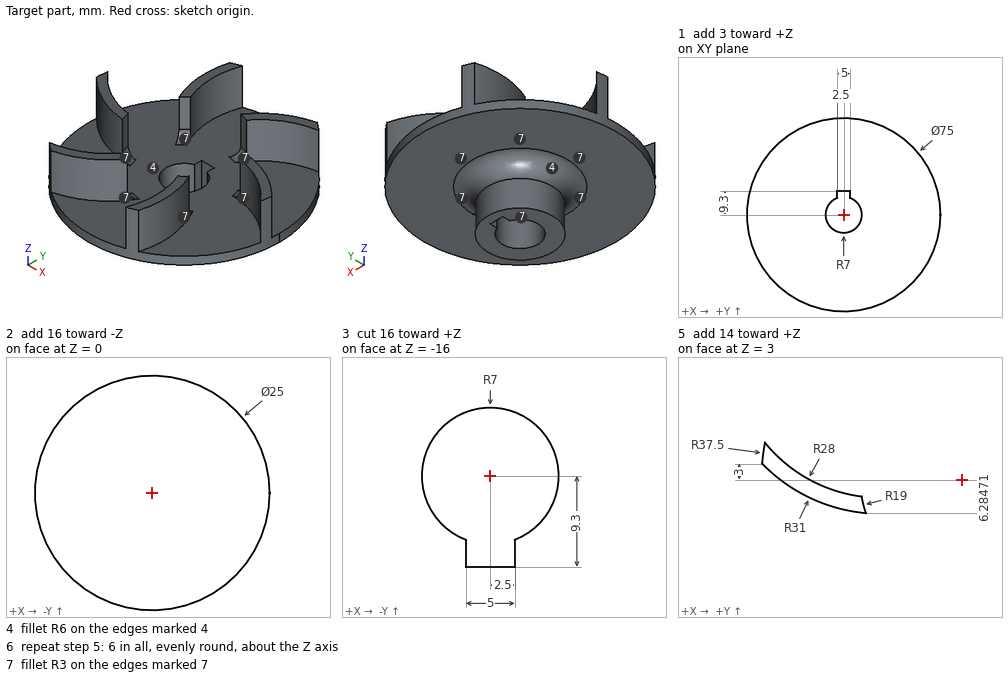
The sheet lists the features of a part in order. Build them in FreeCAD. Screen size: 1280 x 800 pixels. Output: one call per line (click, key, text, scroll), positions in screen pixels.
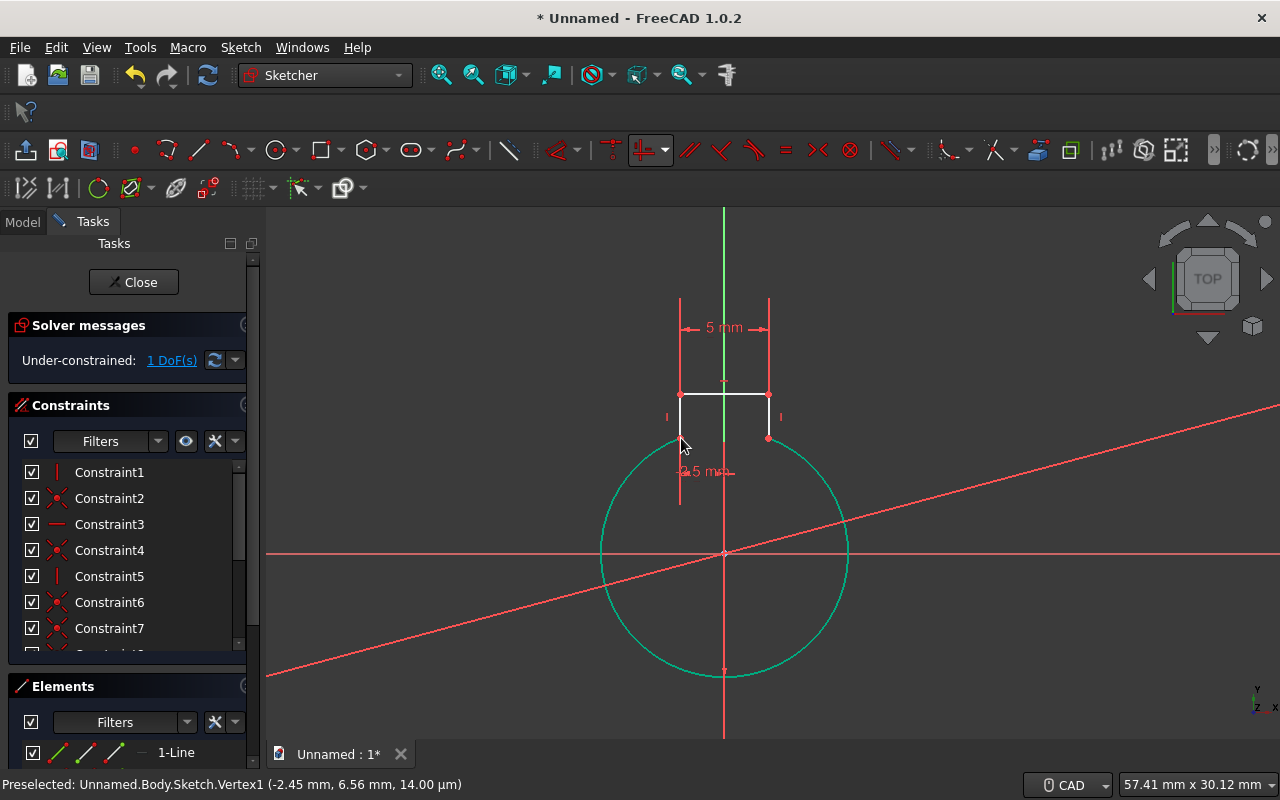
click(680, 394)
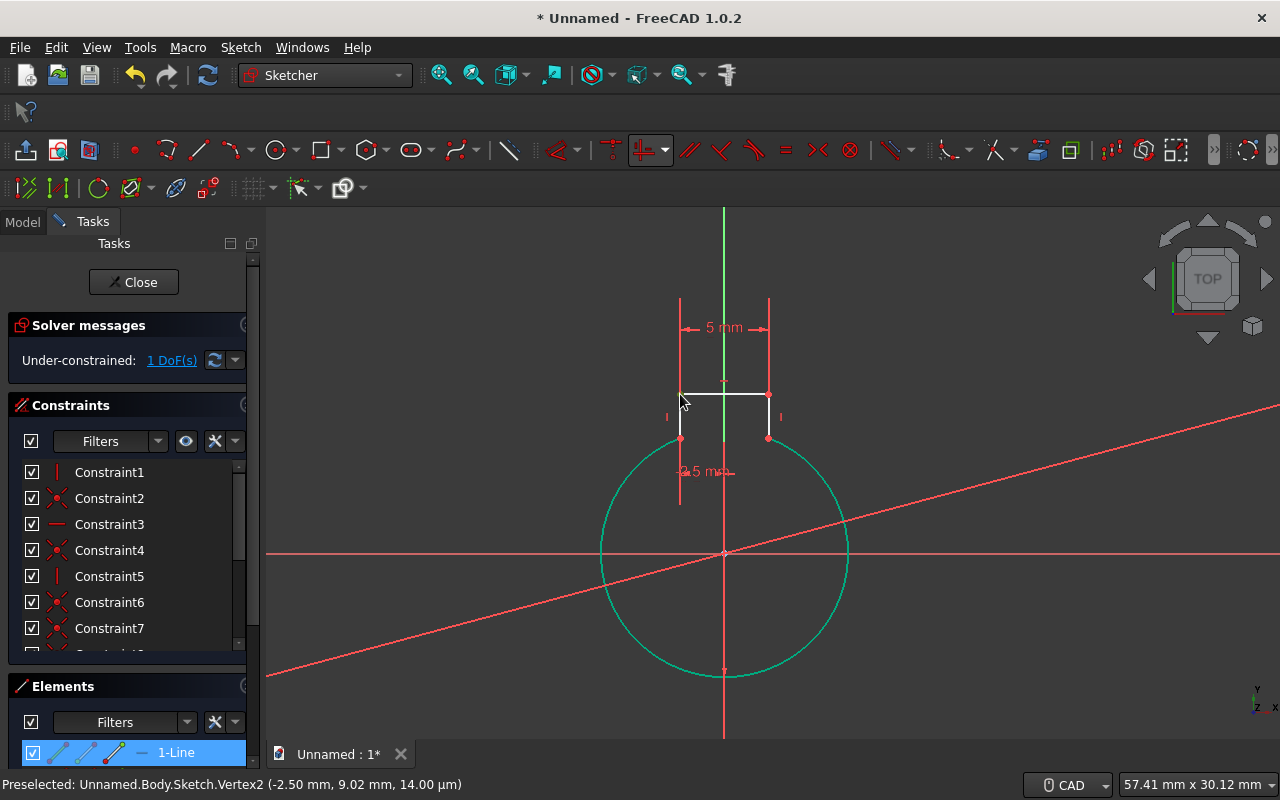
key(i)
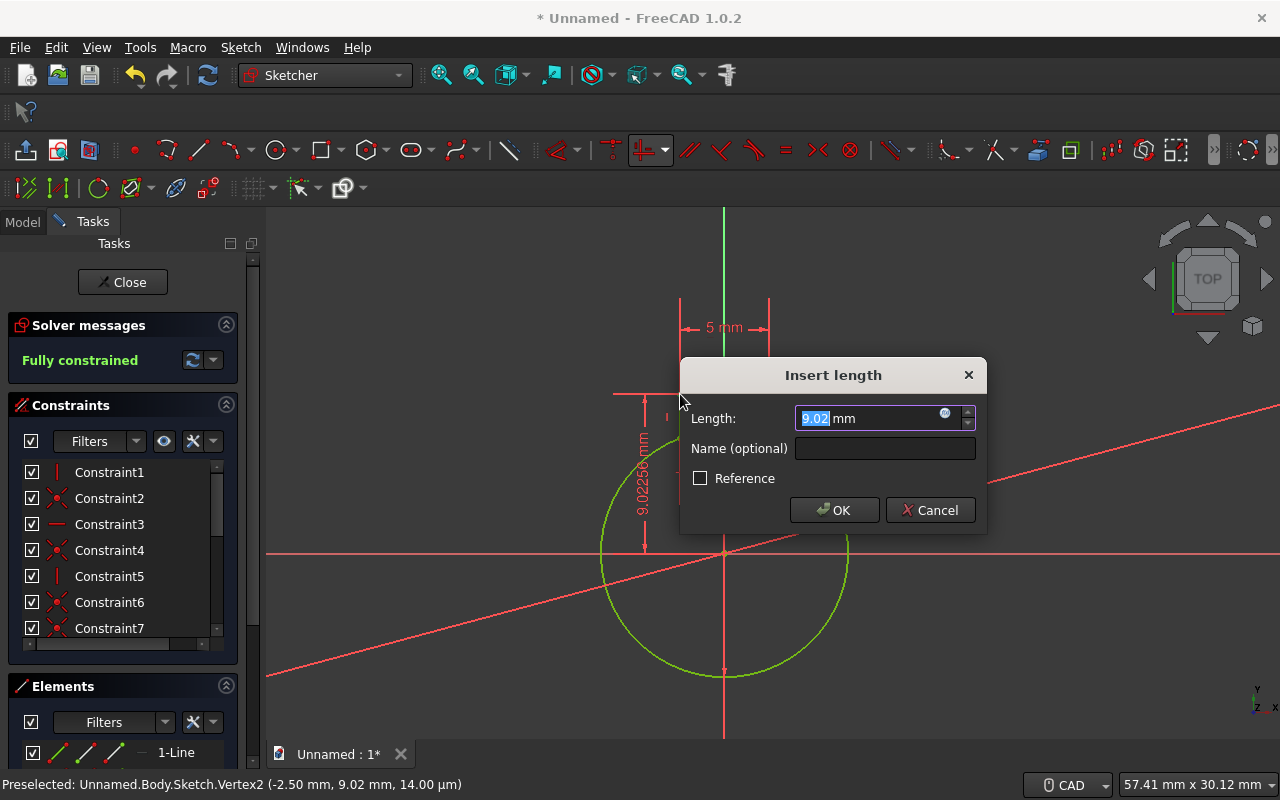
text(9.3)
key(Return)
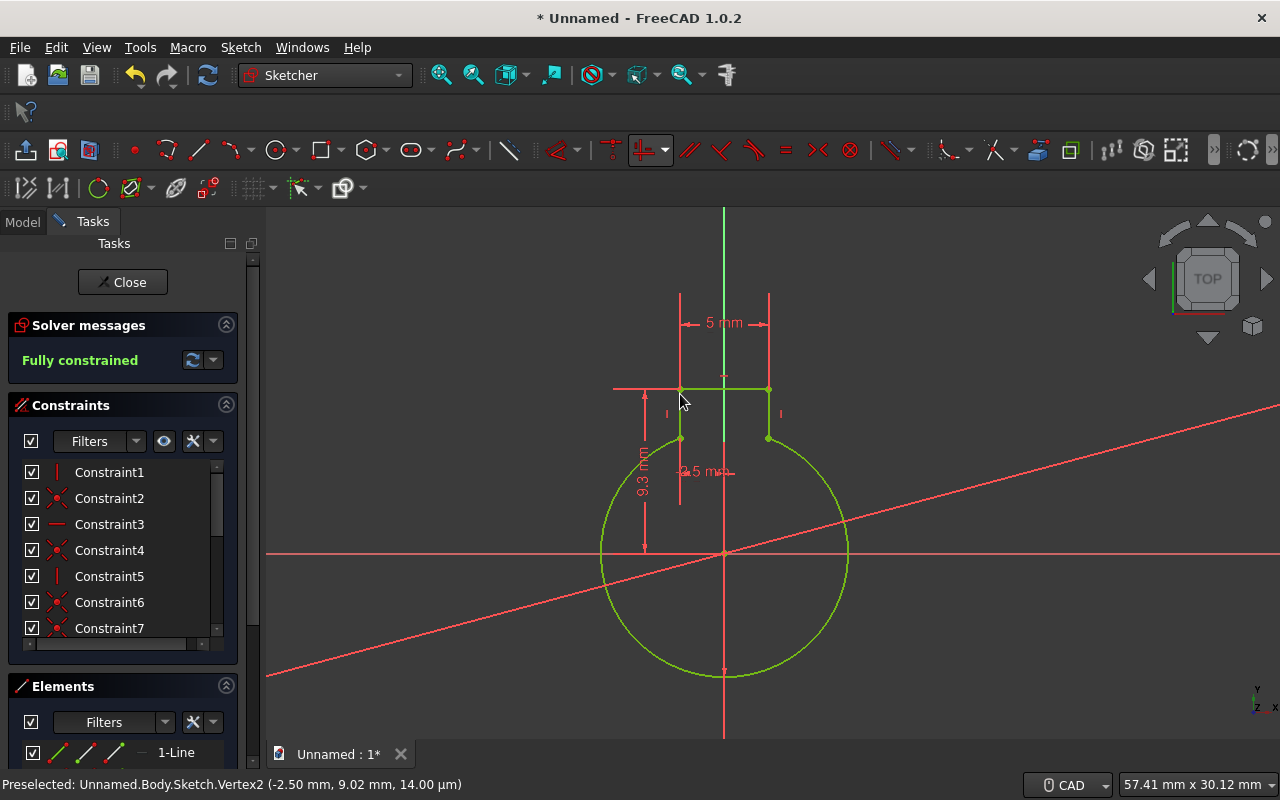
click(123, 282)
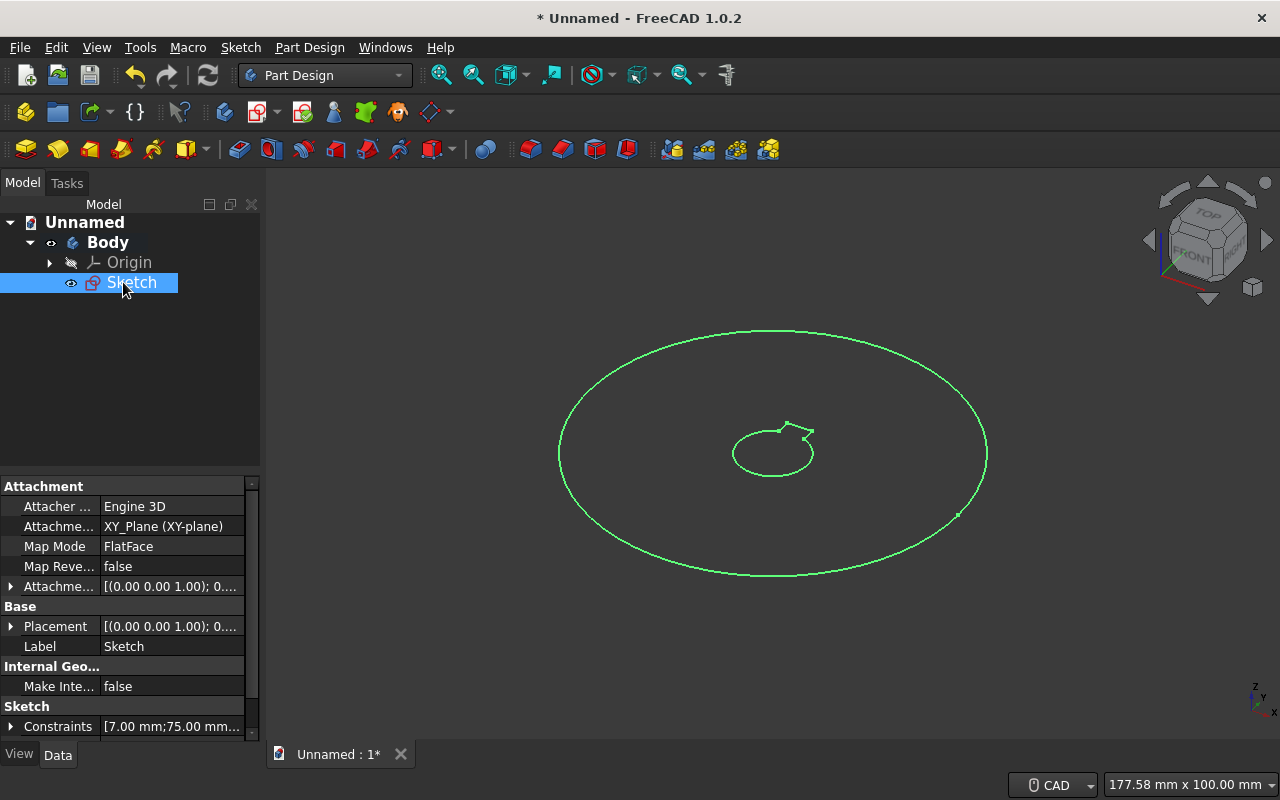
click(26, 150)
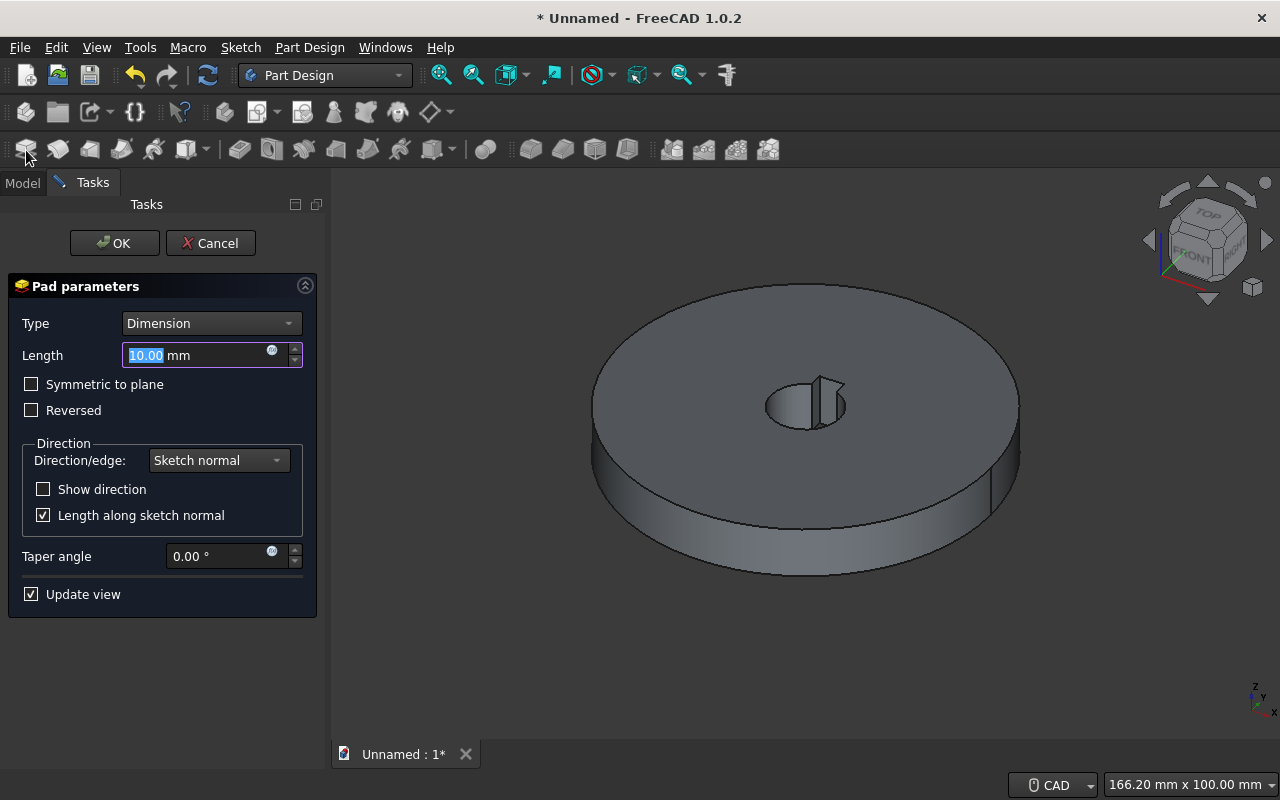
text(3)
key(Tab)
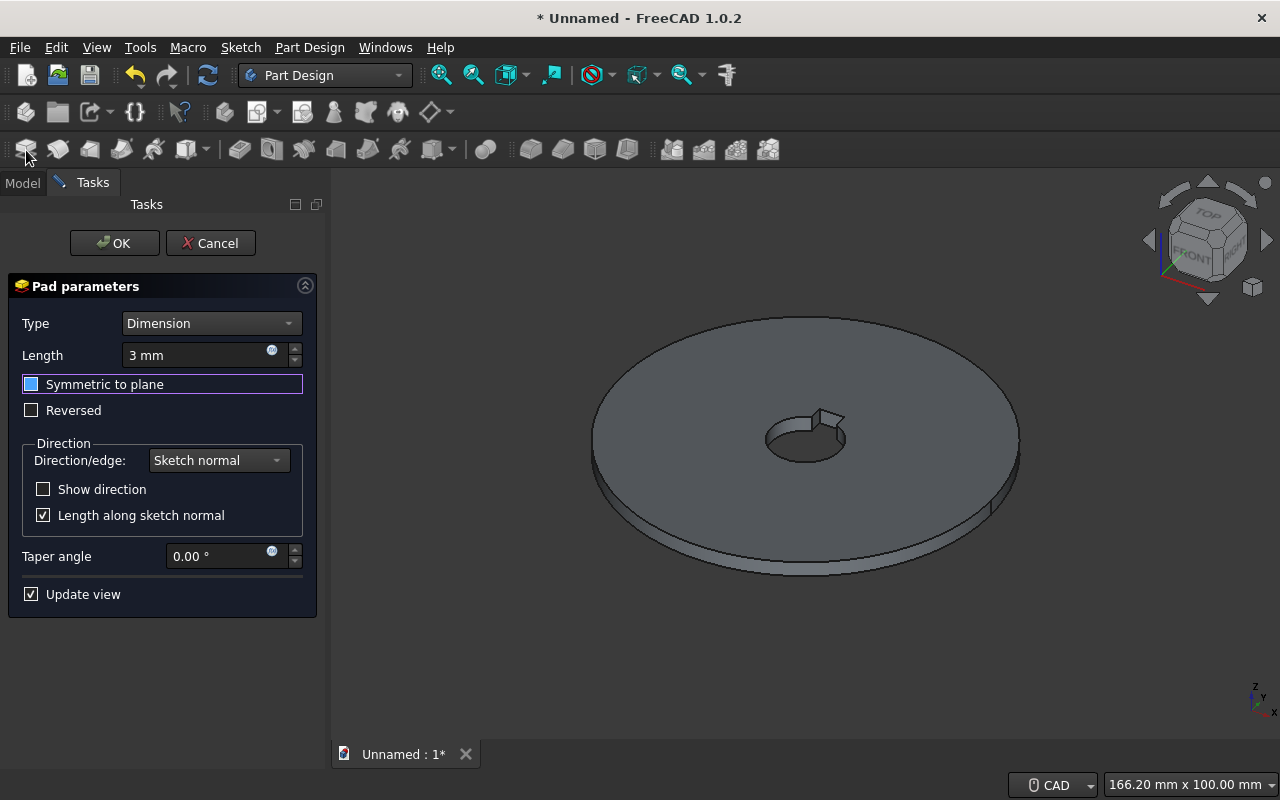
click(115, 243)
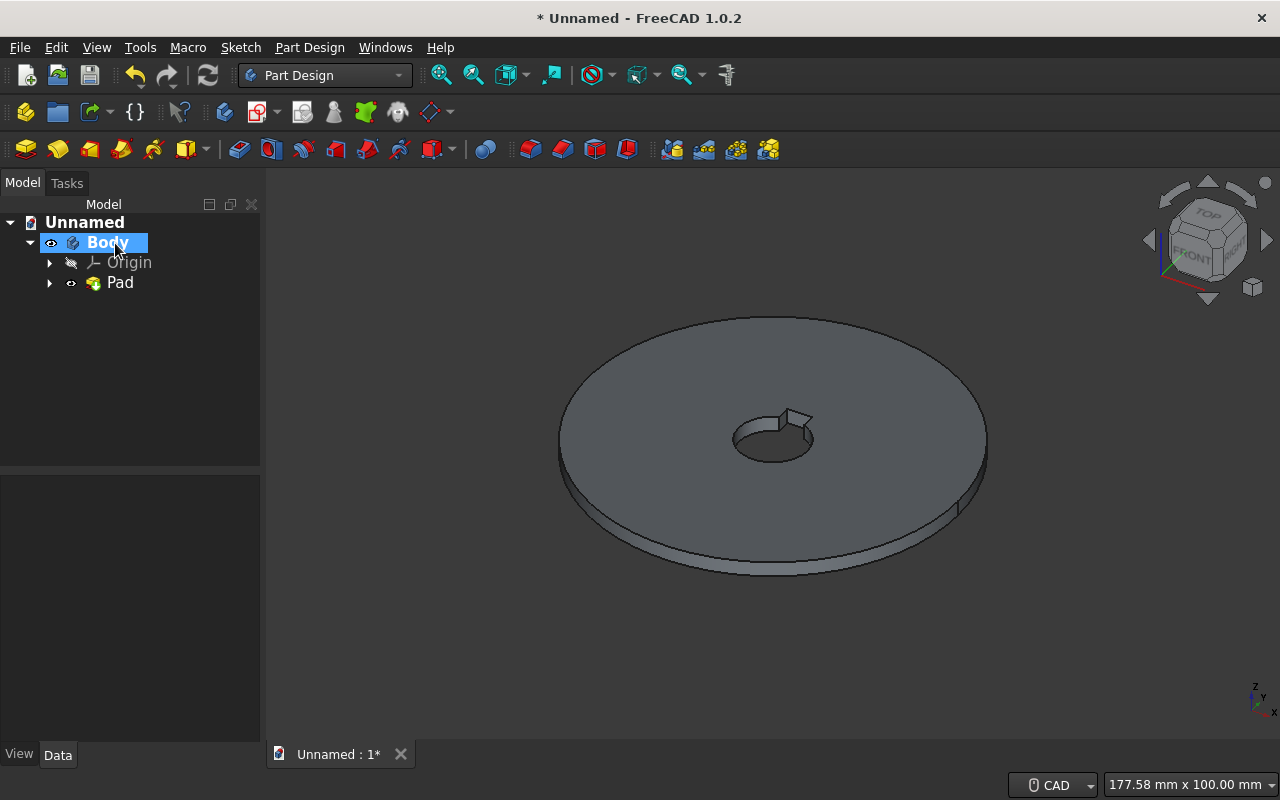
key(5)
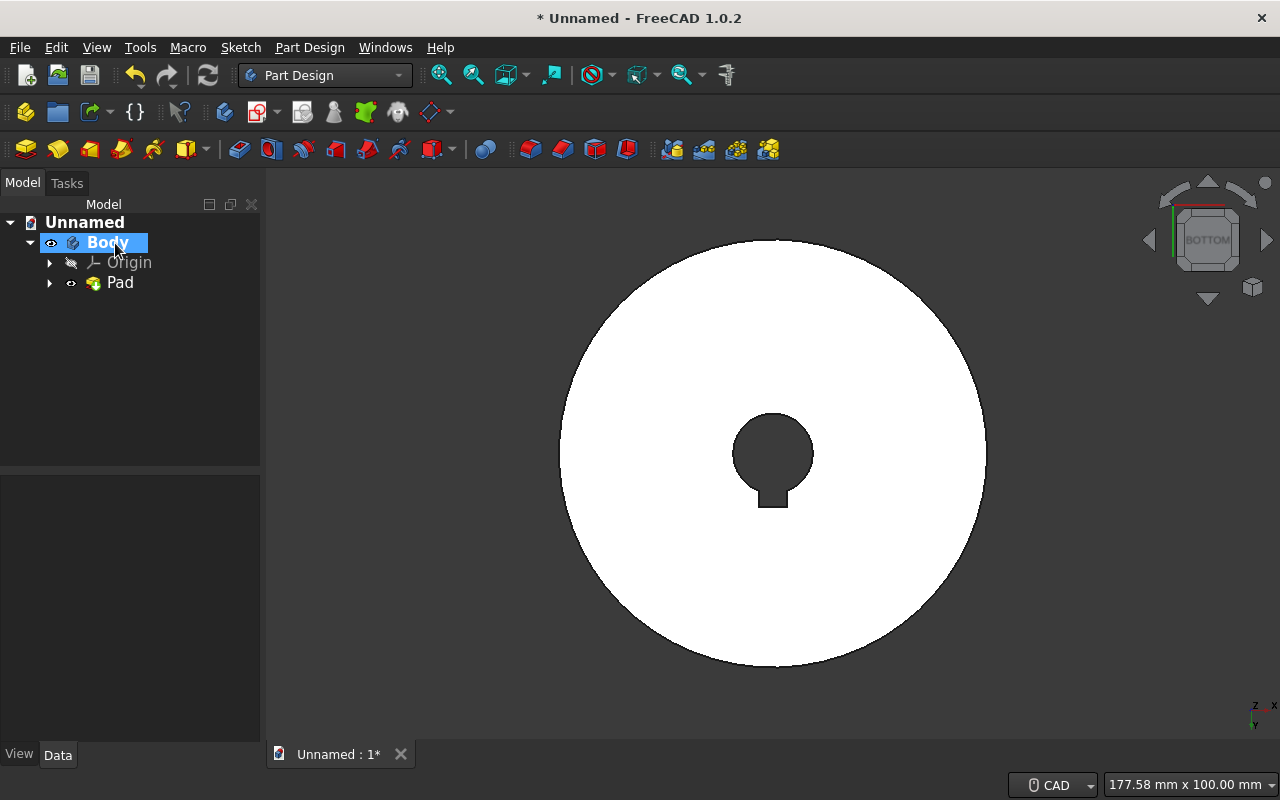
click(651, 452)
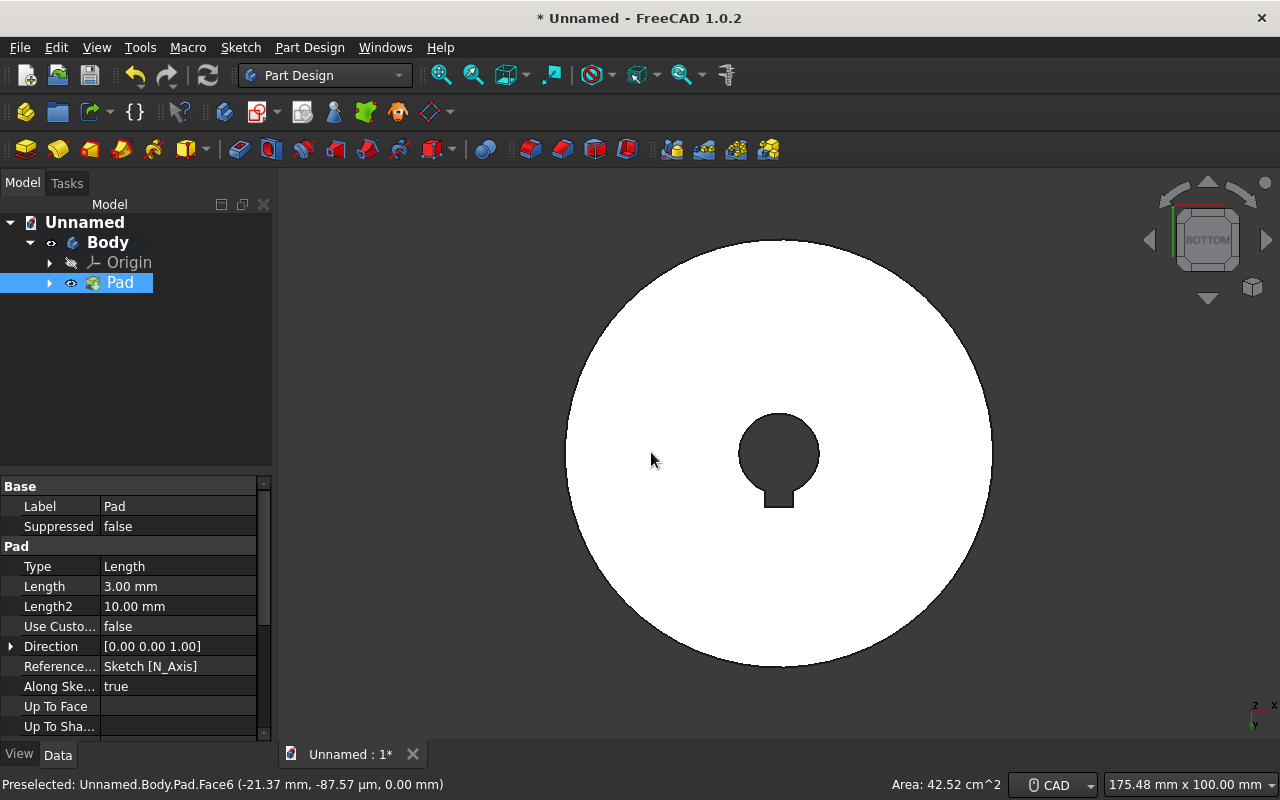
click(258, 112)